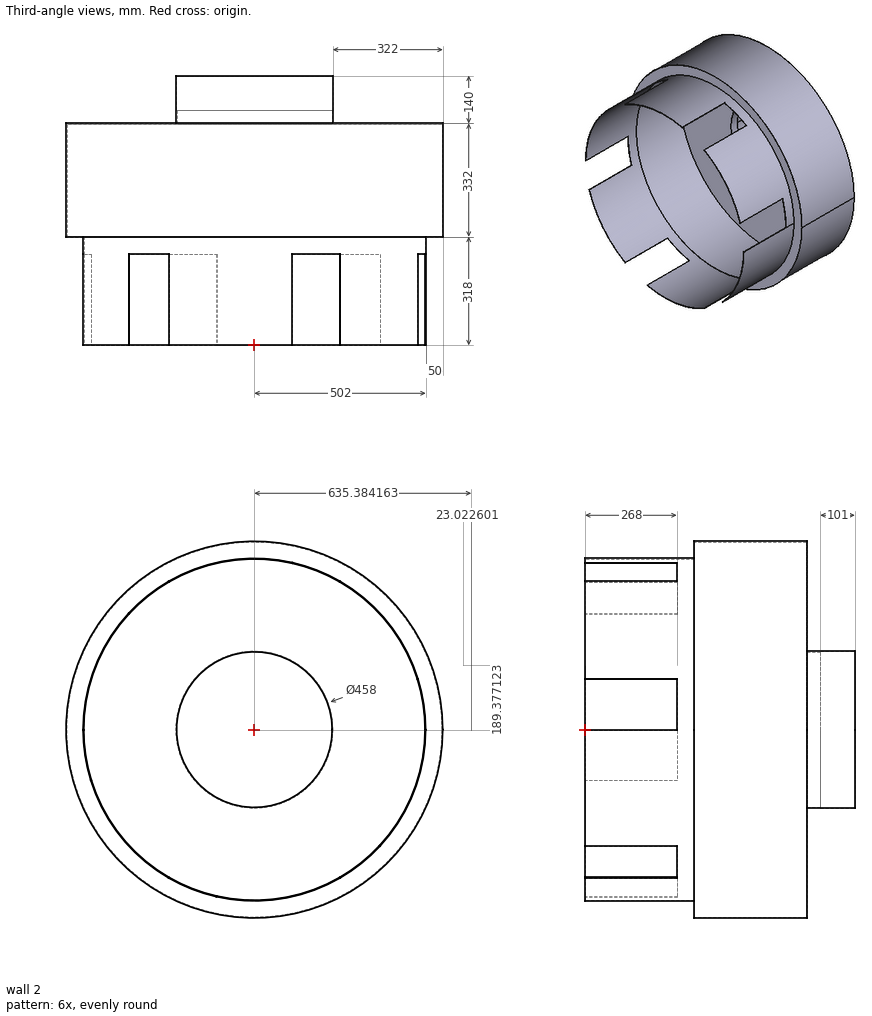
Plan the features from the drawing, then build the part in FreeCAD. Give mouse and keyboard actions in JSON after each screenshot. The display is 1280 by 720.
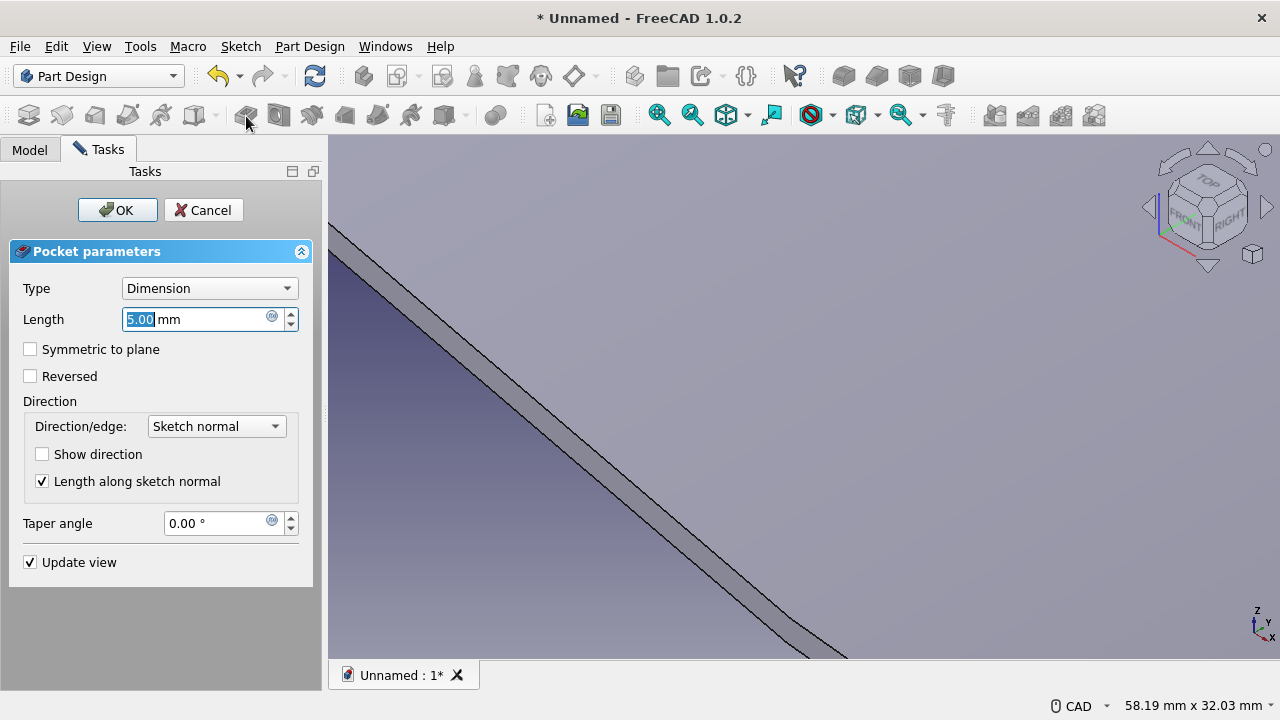
{"action": "type", "text": "268"}
{"action": "key", "text": "Tab"}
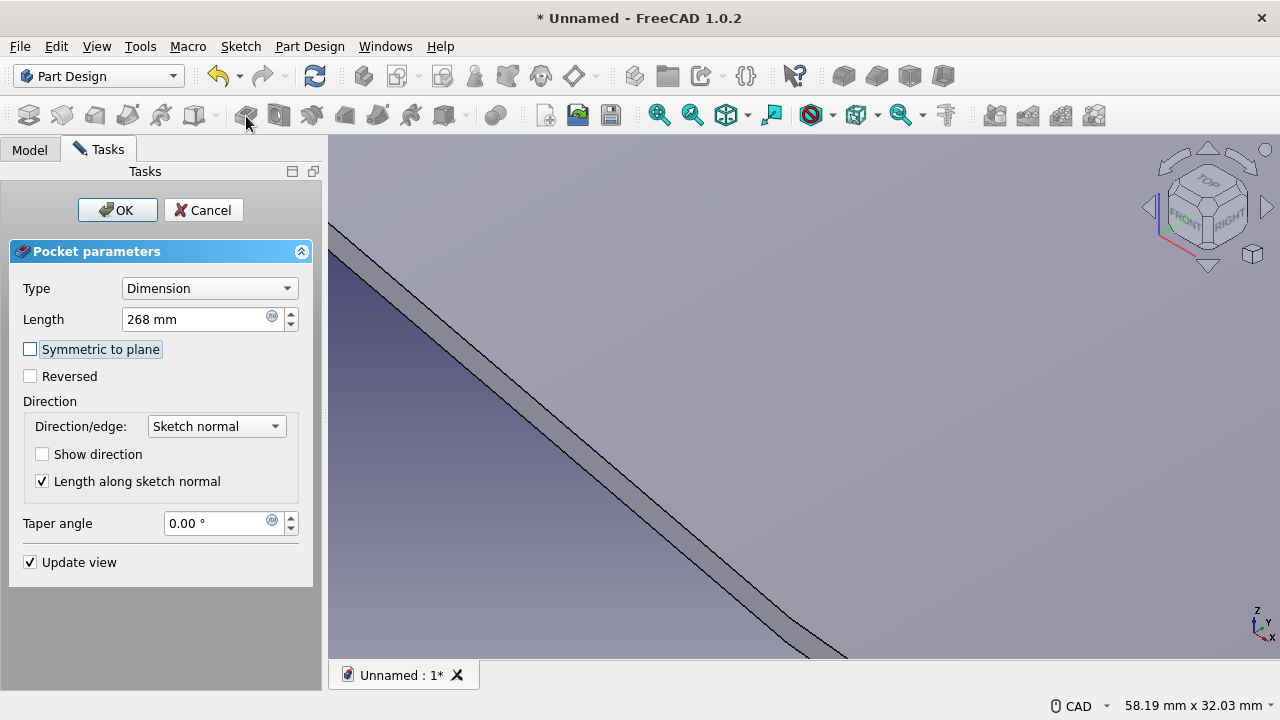
{"action": "left_click", "coordinate": [118, 210]}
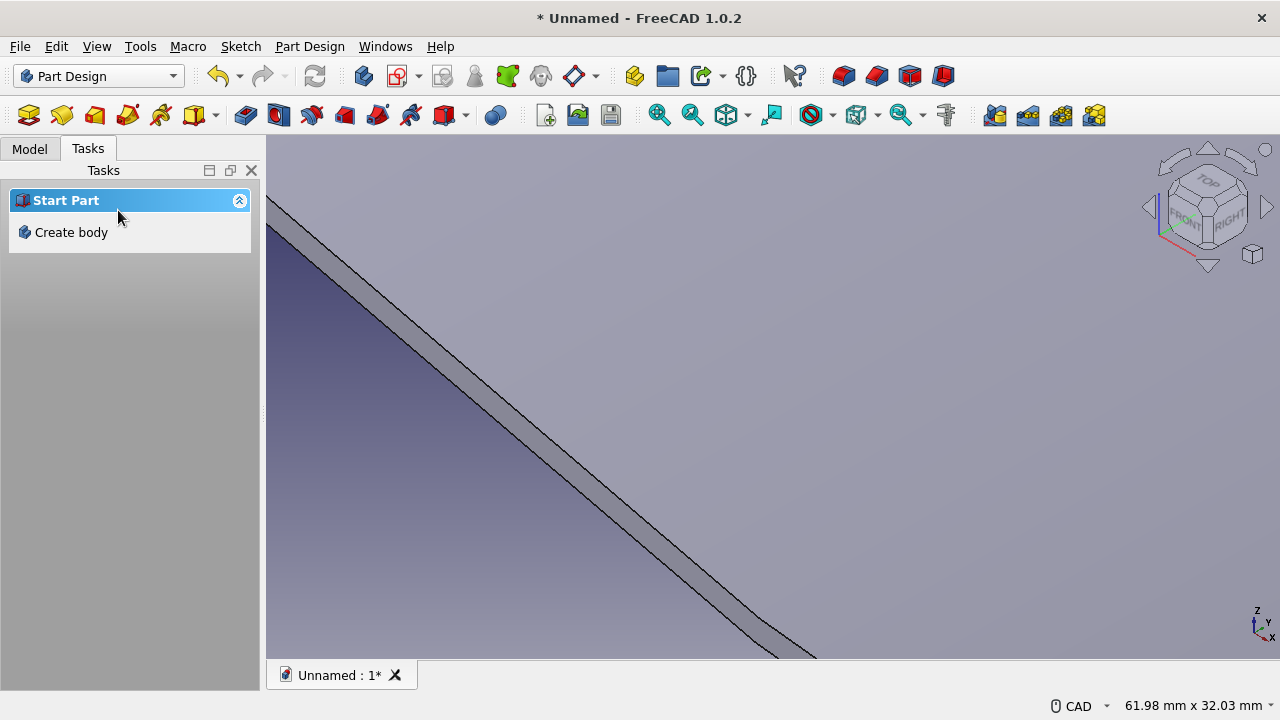
{"action": "left_click", "coordinate": [660, 116]}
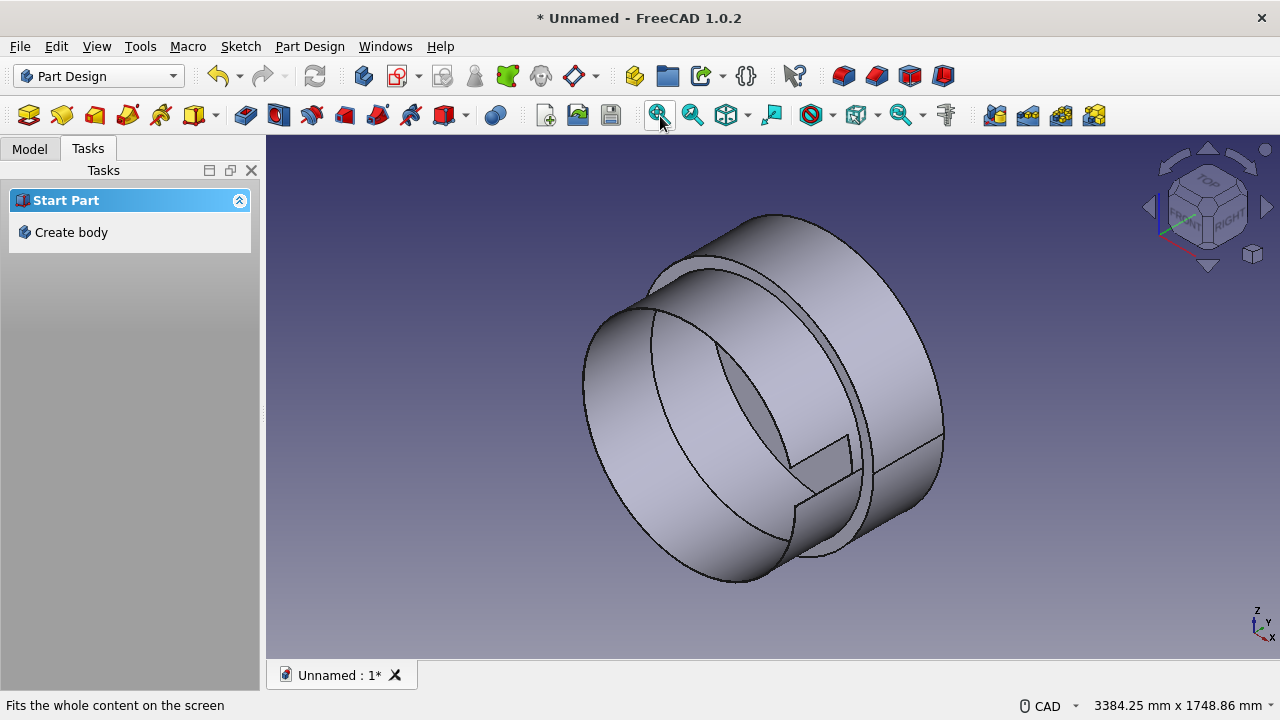
{"action": "left_click", "coordinate": [30, 148]}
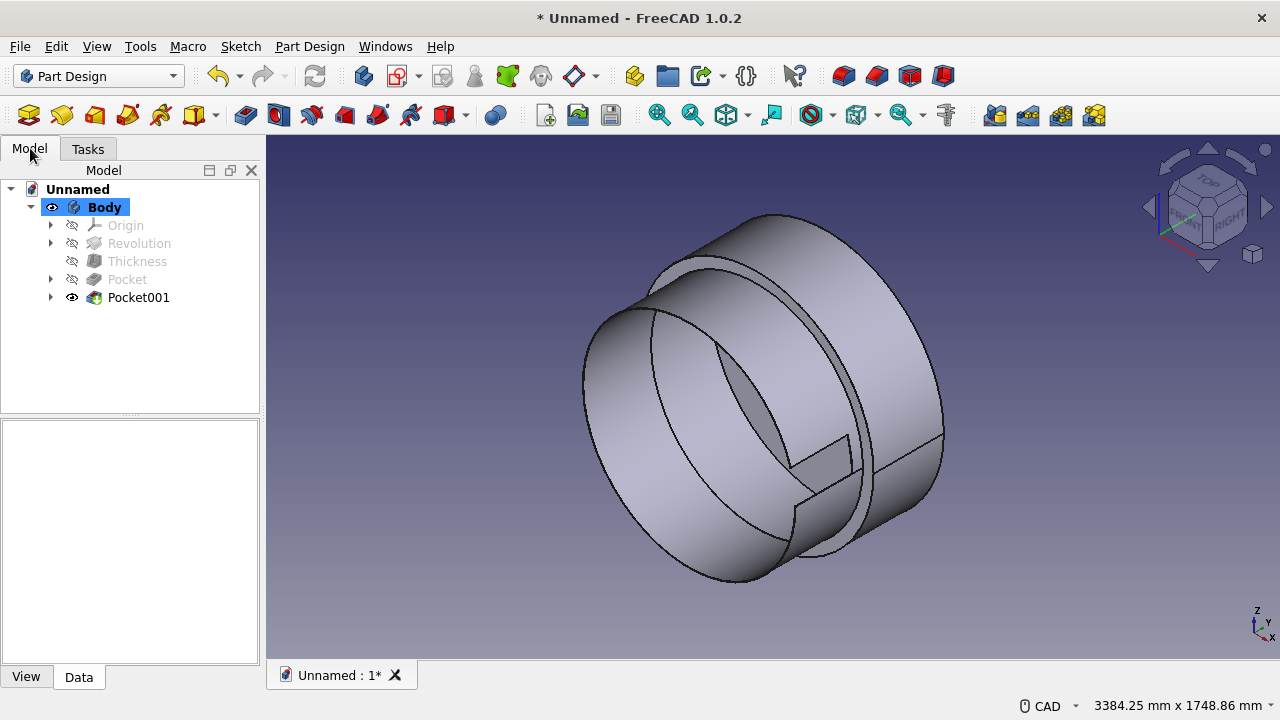
{"action": "left_click", "coordinate": [117, 297]}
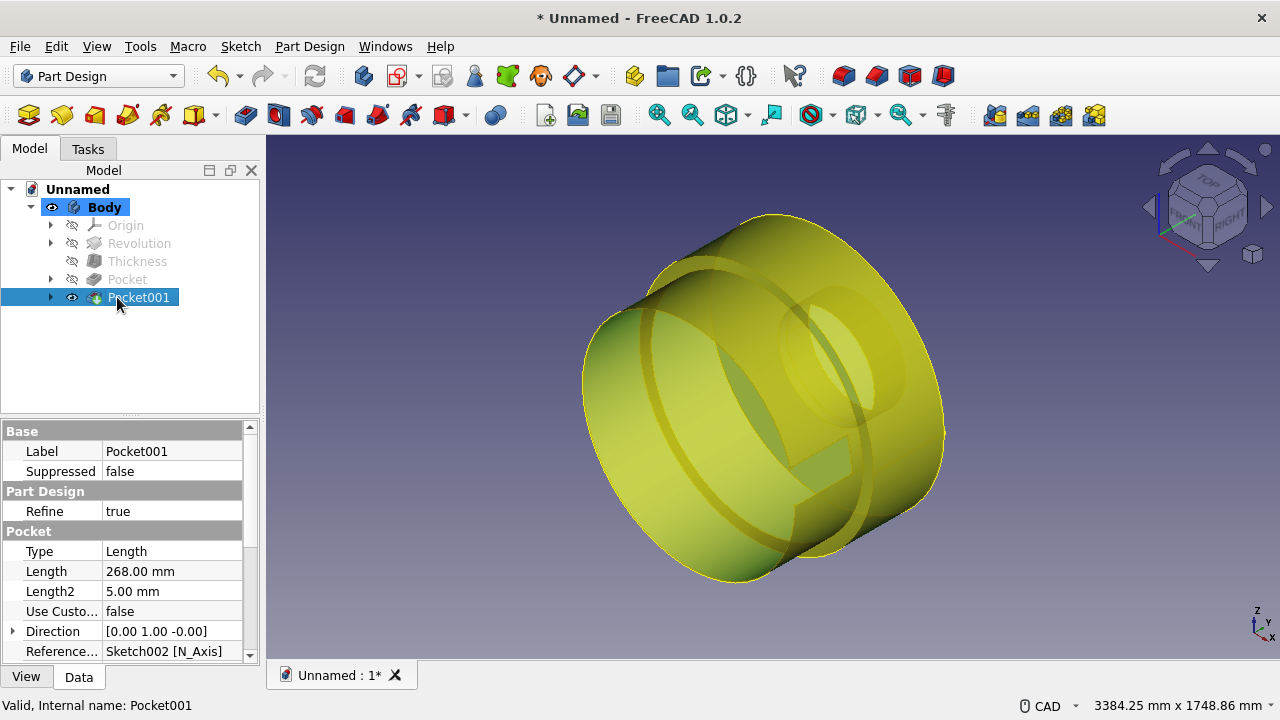
{"action": "left_click", "coordinate": [1061, 116]}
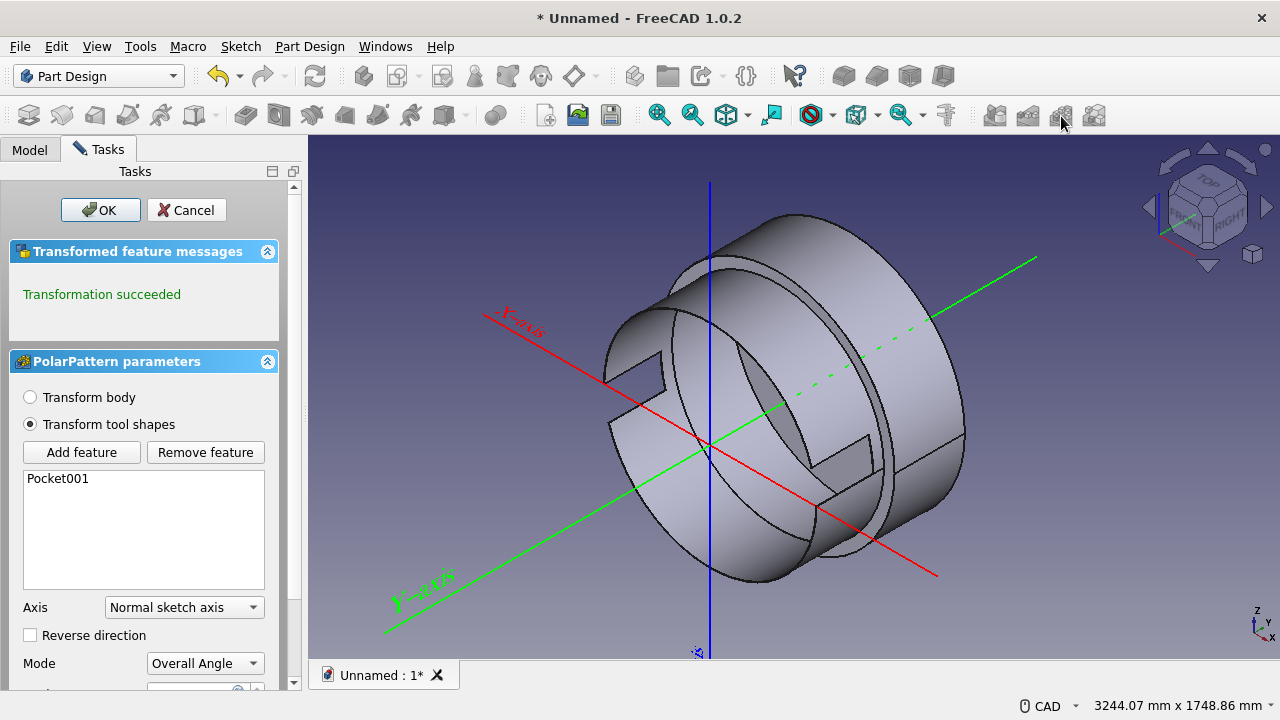
{"action": "left_click", "coordinate": [185, 608]}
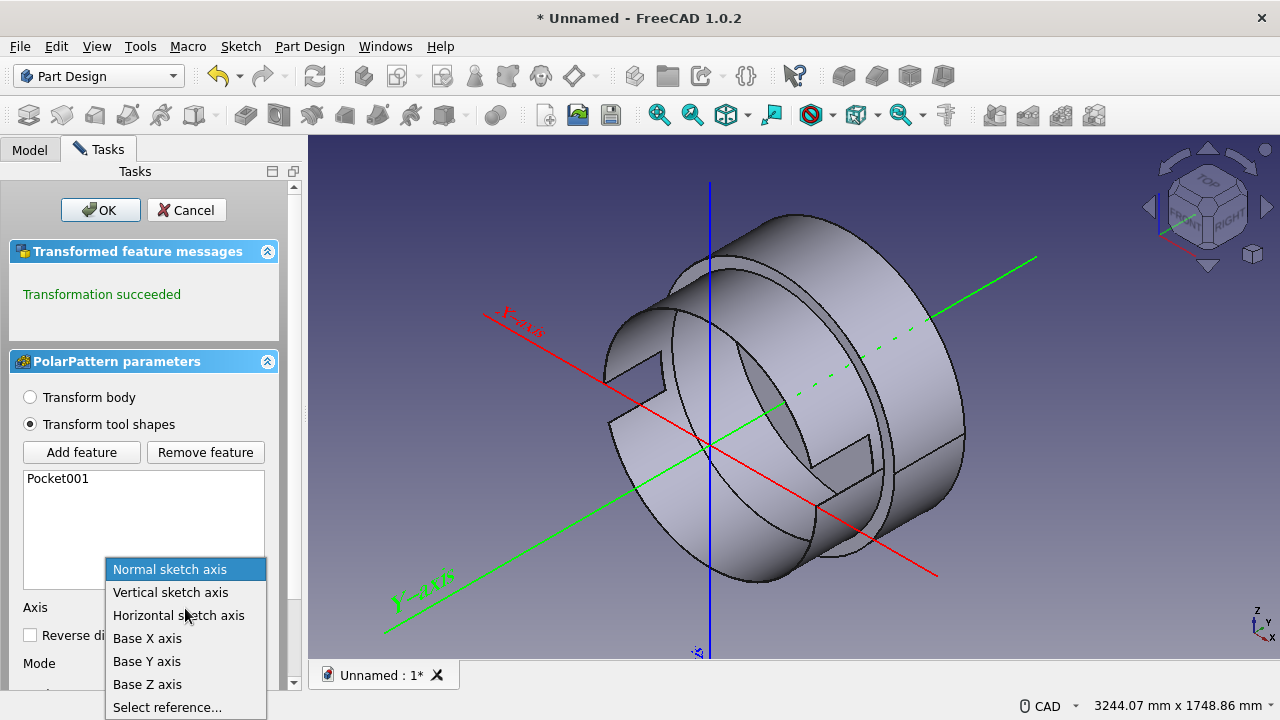
{"action": "left_click", "coordinate": [184, 662]}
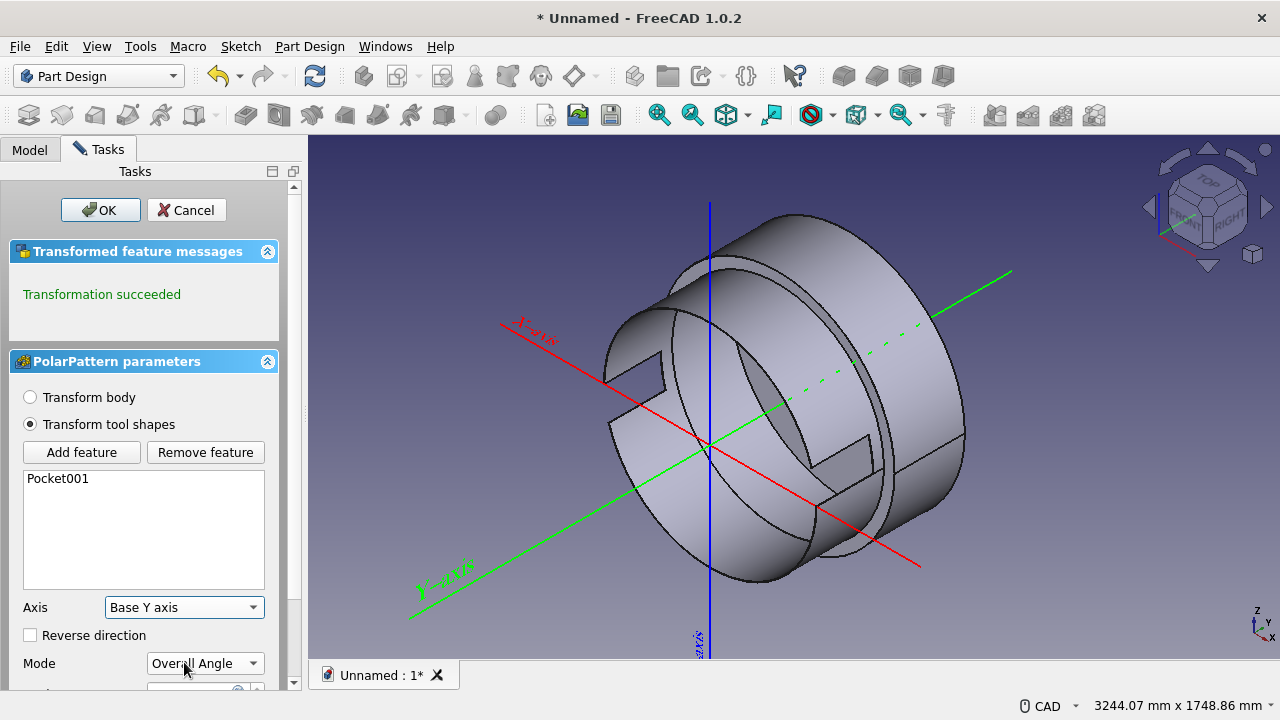
{"action": "scroll", "coordinate": [294, 436], "scroll_direction": "down", "scroll_amount": 2}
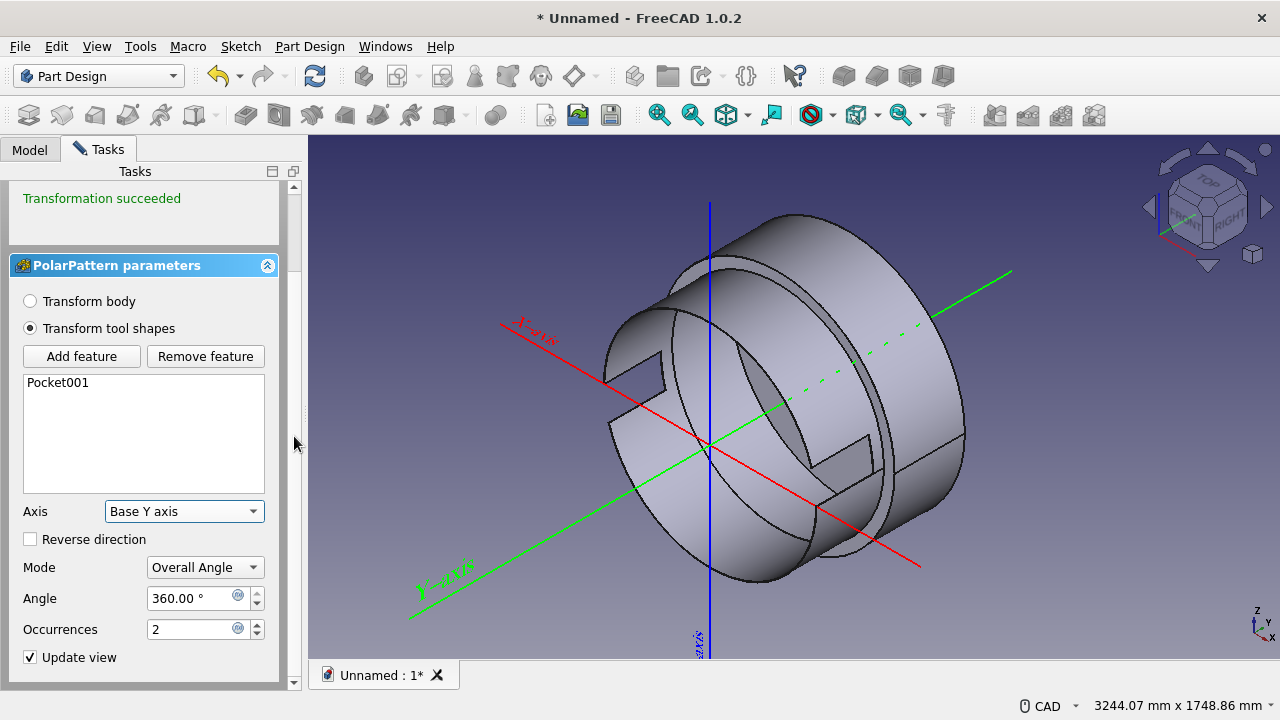
{"action": "triple_click", "coordinate": [199, 630]}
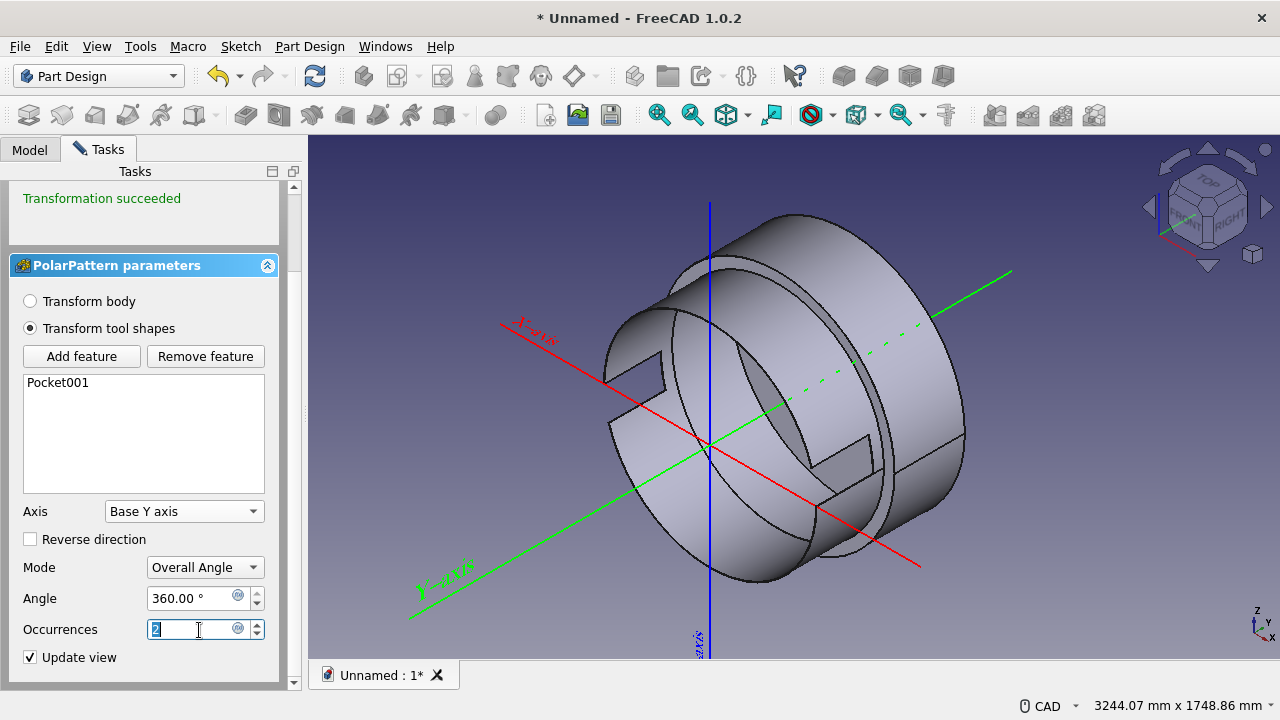
{"action": "type", "text": "6"}
{"action": "key", "text": "Tab"}